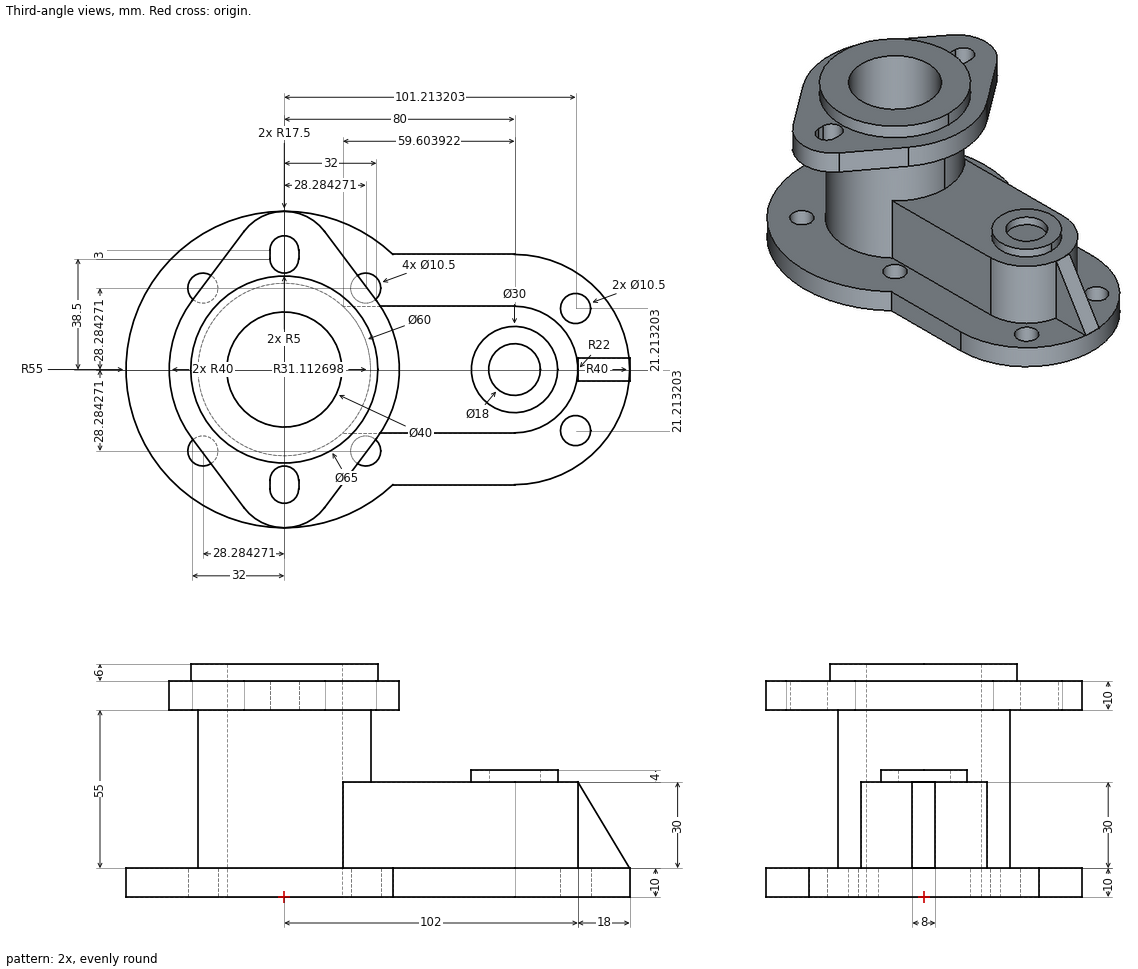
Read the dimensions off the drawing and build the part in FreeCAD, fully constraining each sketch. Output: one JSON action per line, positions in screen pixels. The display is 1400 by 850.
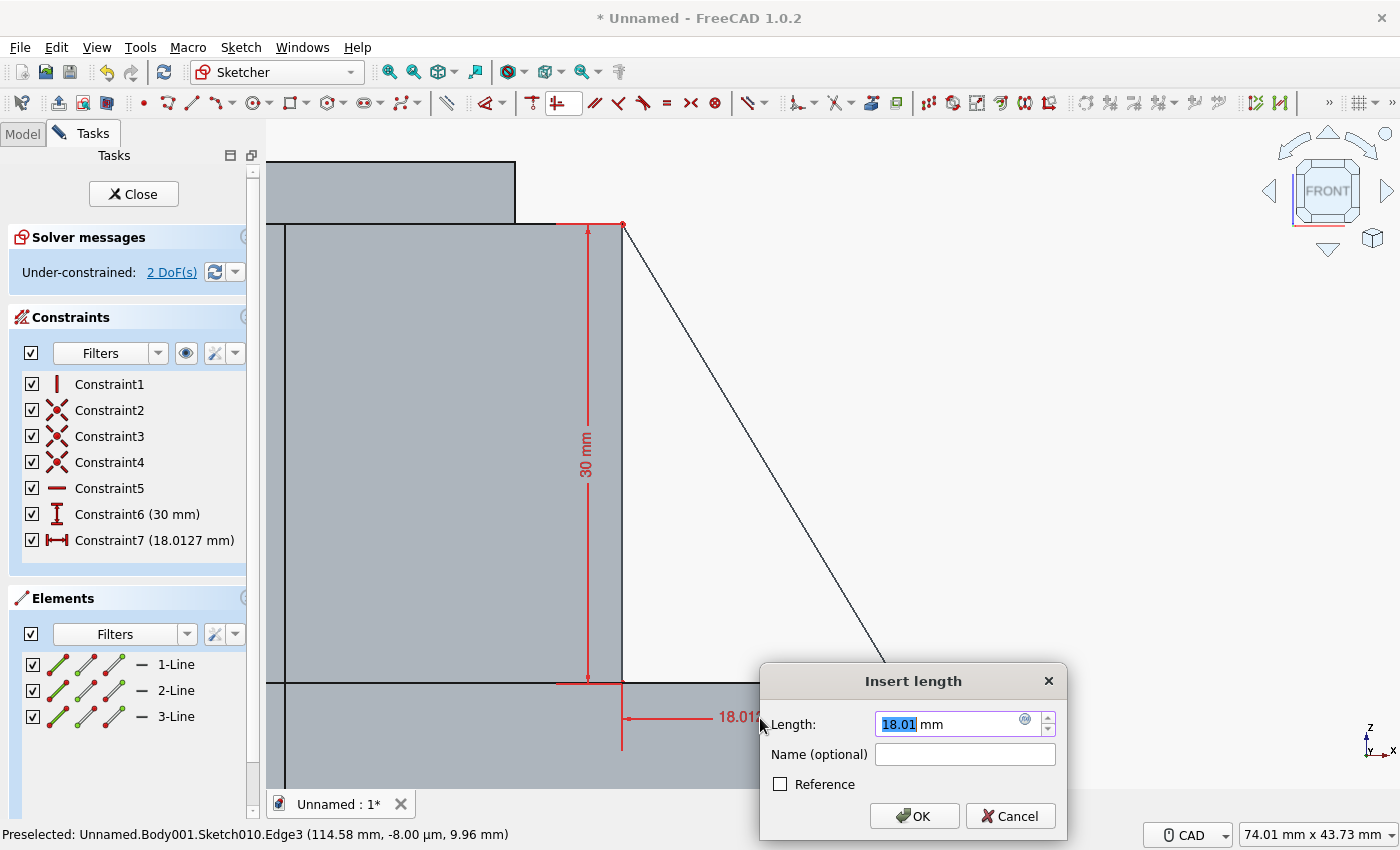
{"action": "type", "text": "18"}
{"action": "key", "text": "Return"}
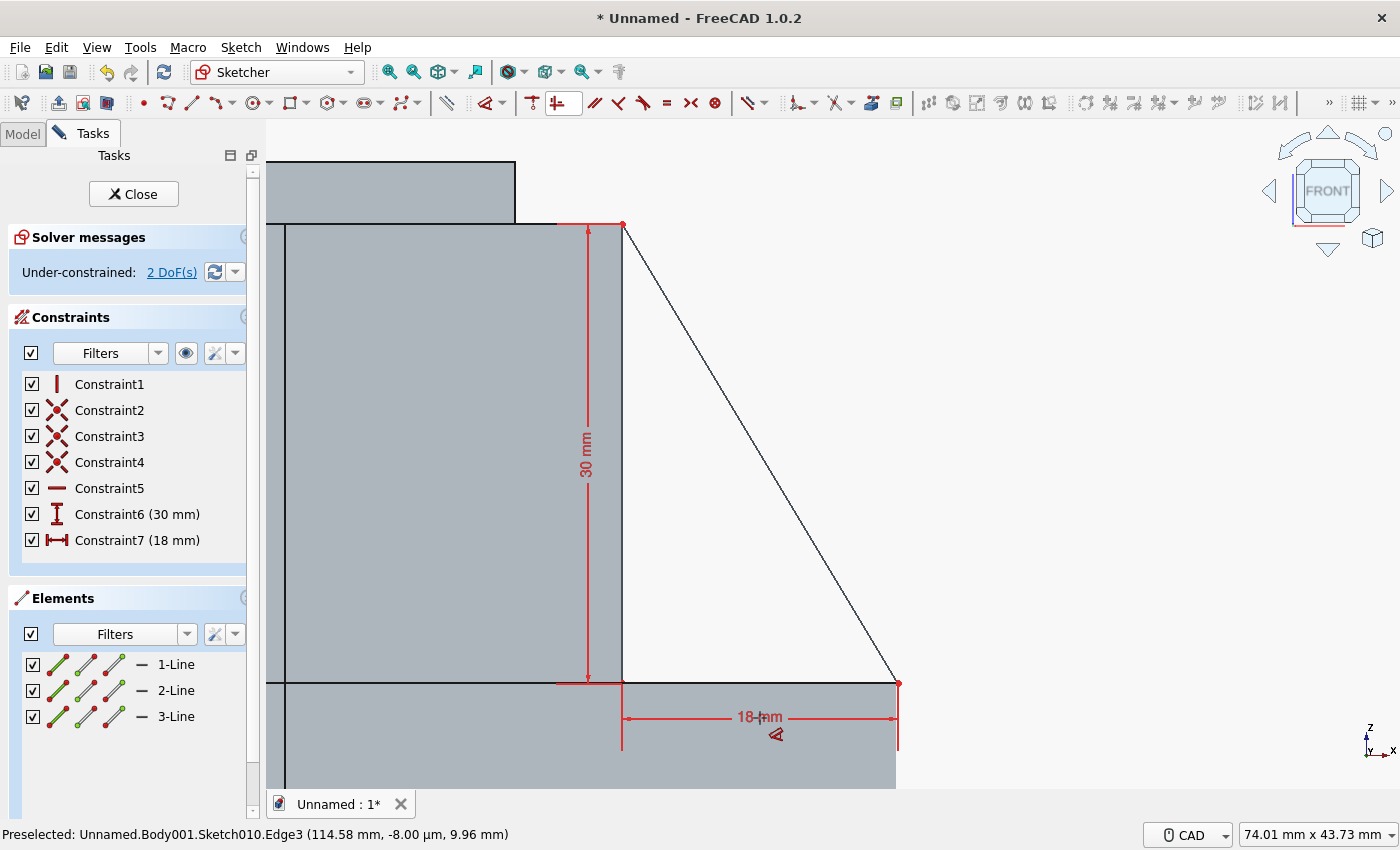
{"action": "left_click", "coordinate": [622, 684]}
{"action": "left_click", "coordinate": [656, 722]}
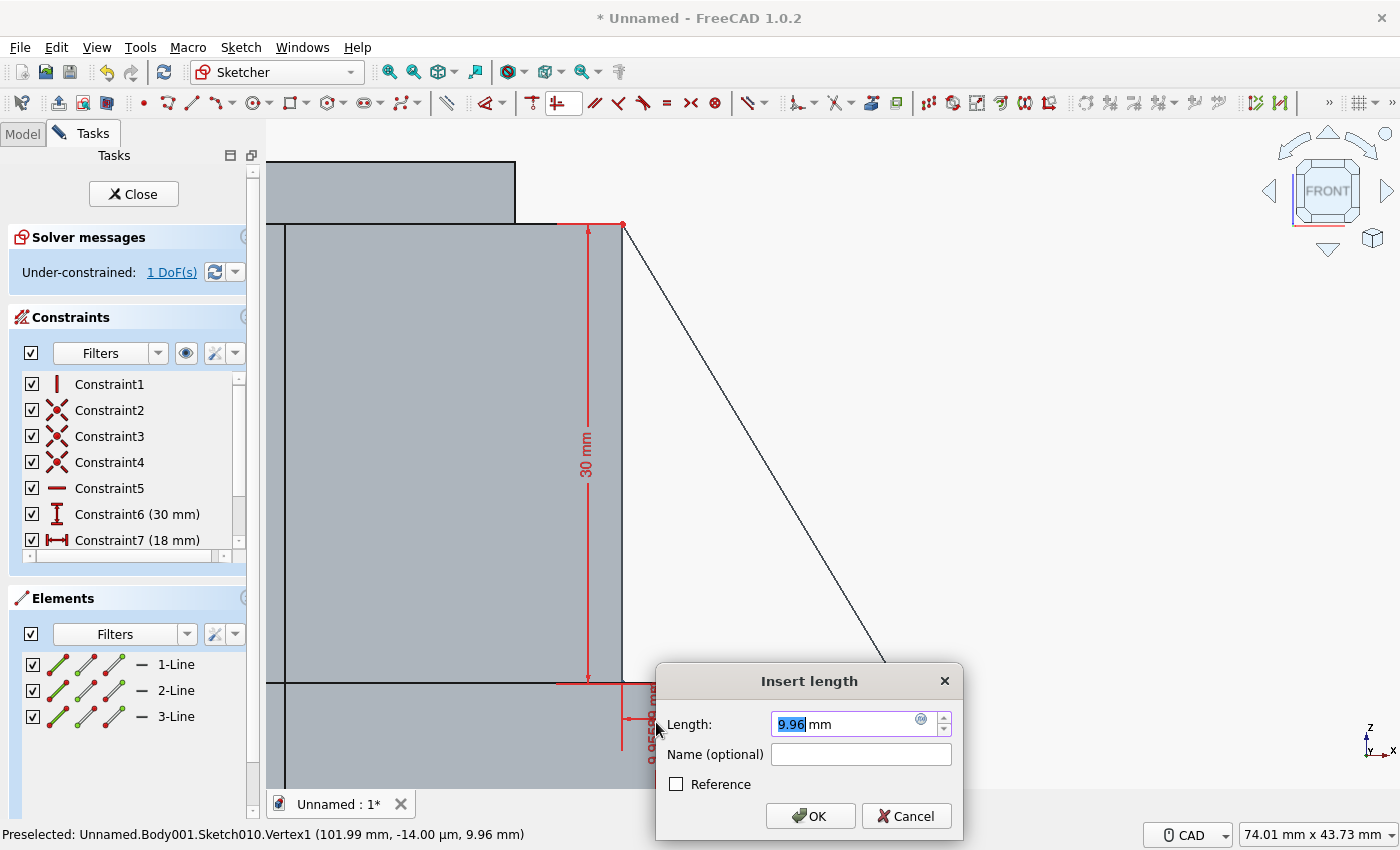
{"action": "type", "text": "10"}
{"action": "key", "text": "Return"}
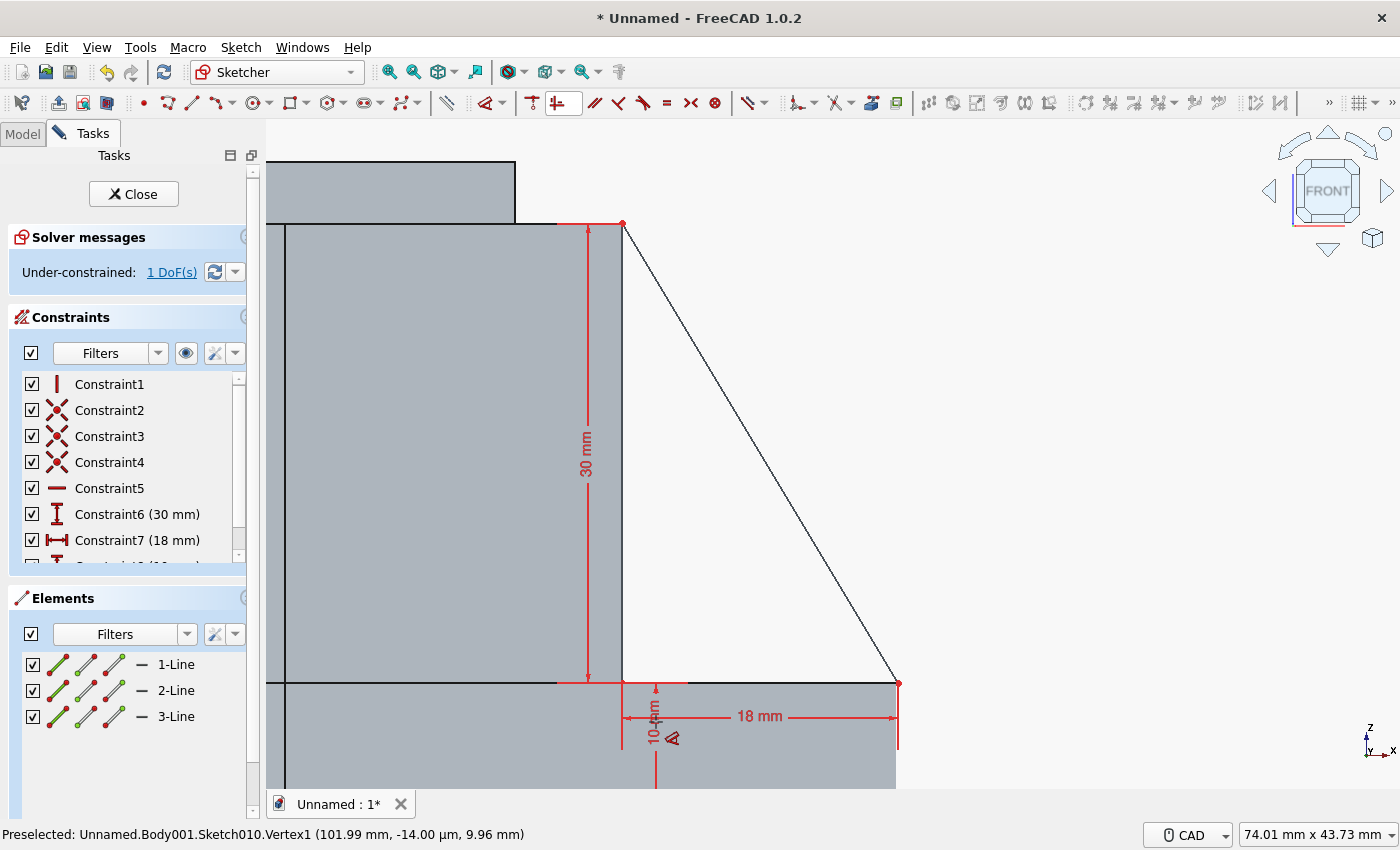
{"action": "left_click", "coordinate": [622, 683]}
{"action": "left_click", "coordinate": [458, 649]}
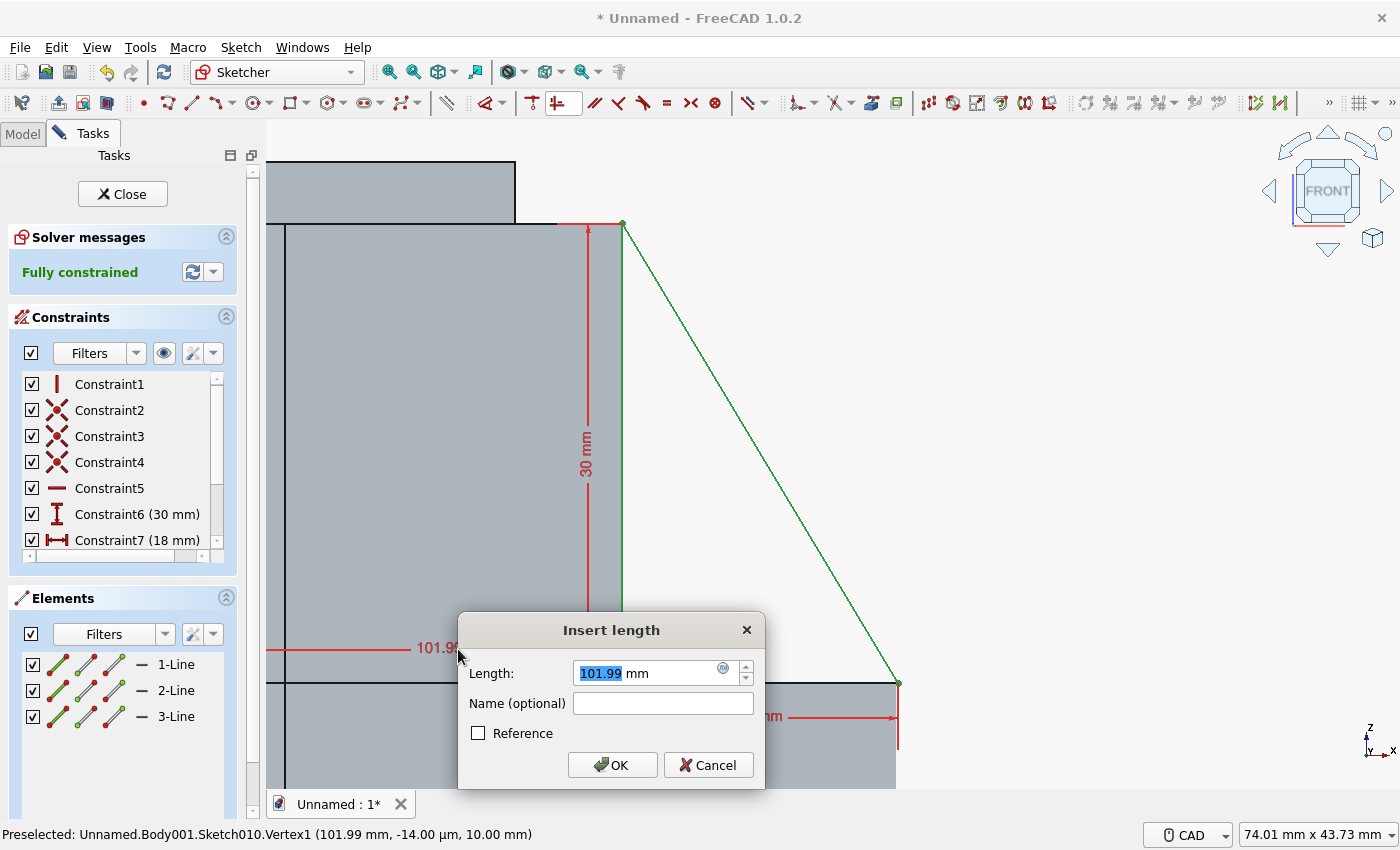
{"action": "type", "text": "102"}
{"action": "key", "text": "Return"}
{"action": "key", "text": "Escape"}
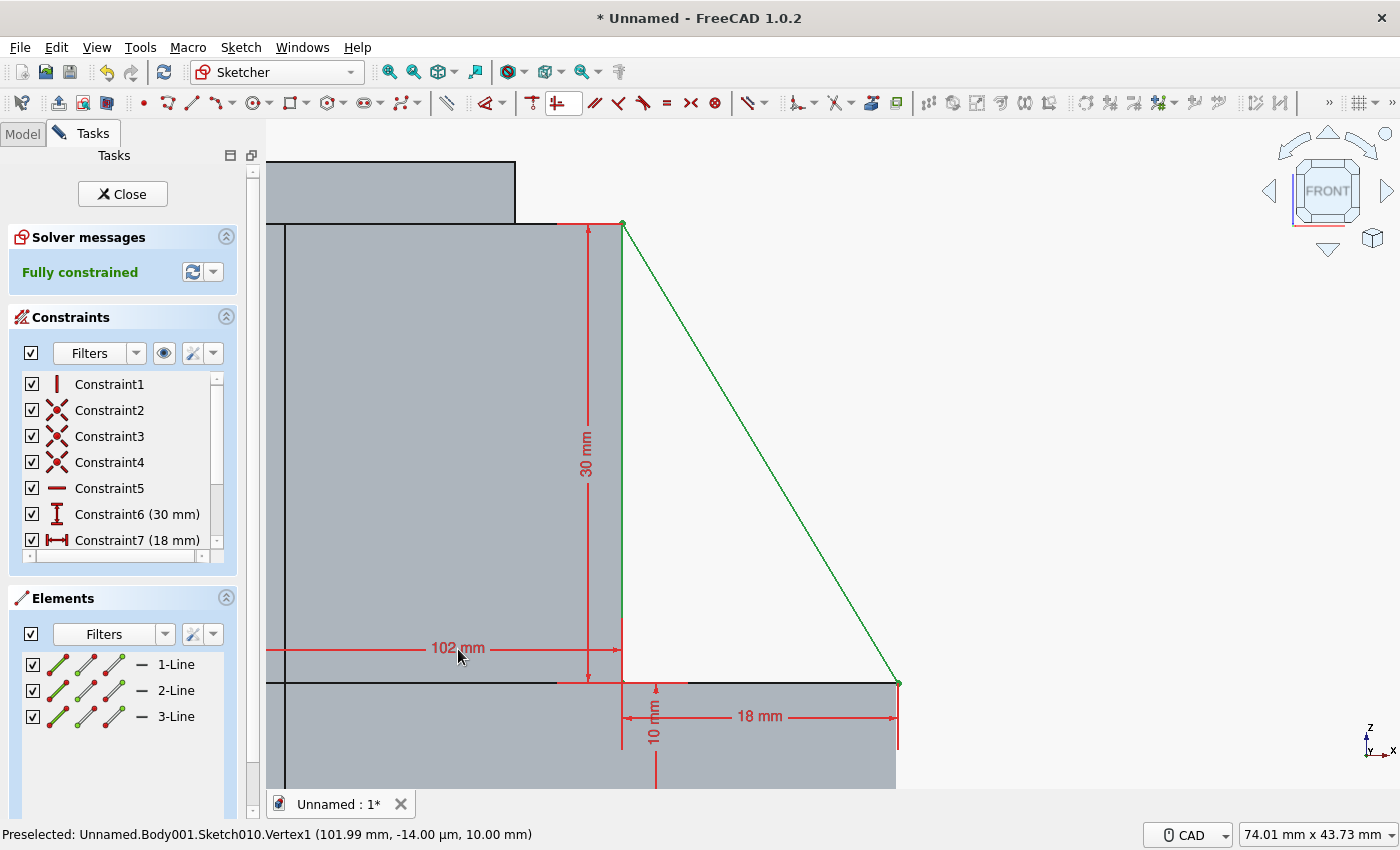
{"action": "left_click", "coordinate": [123, 194]}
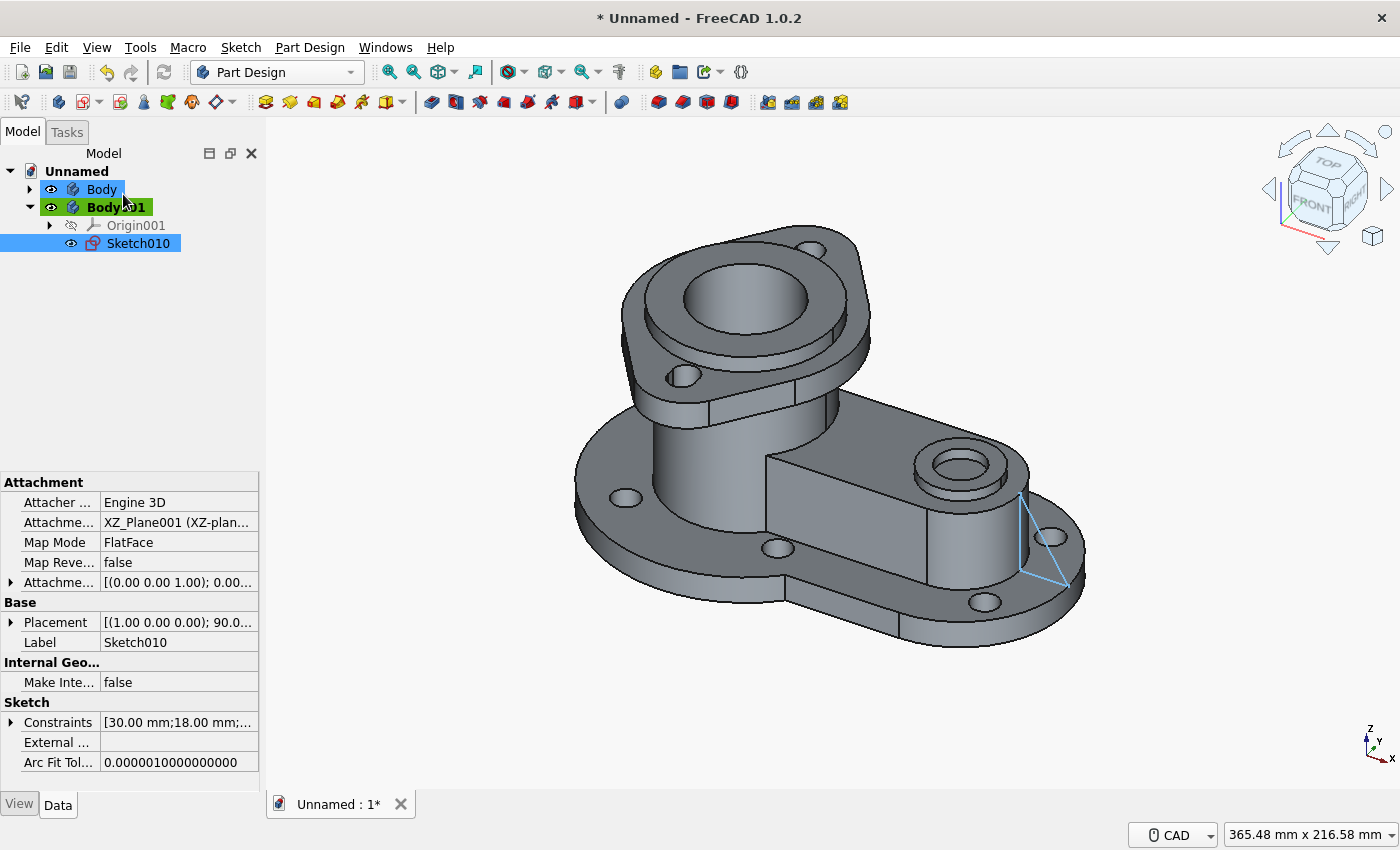
{"action": "left_click", "coordinate": [266, 102]}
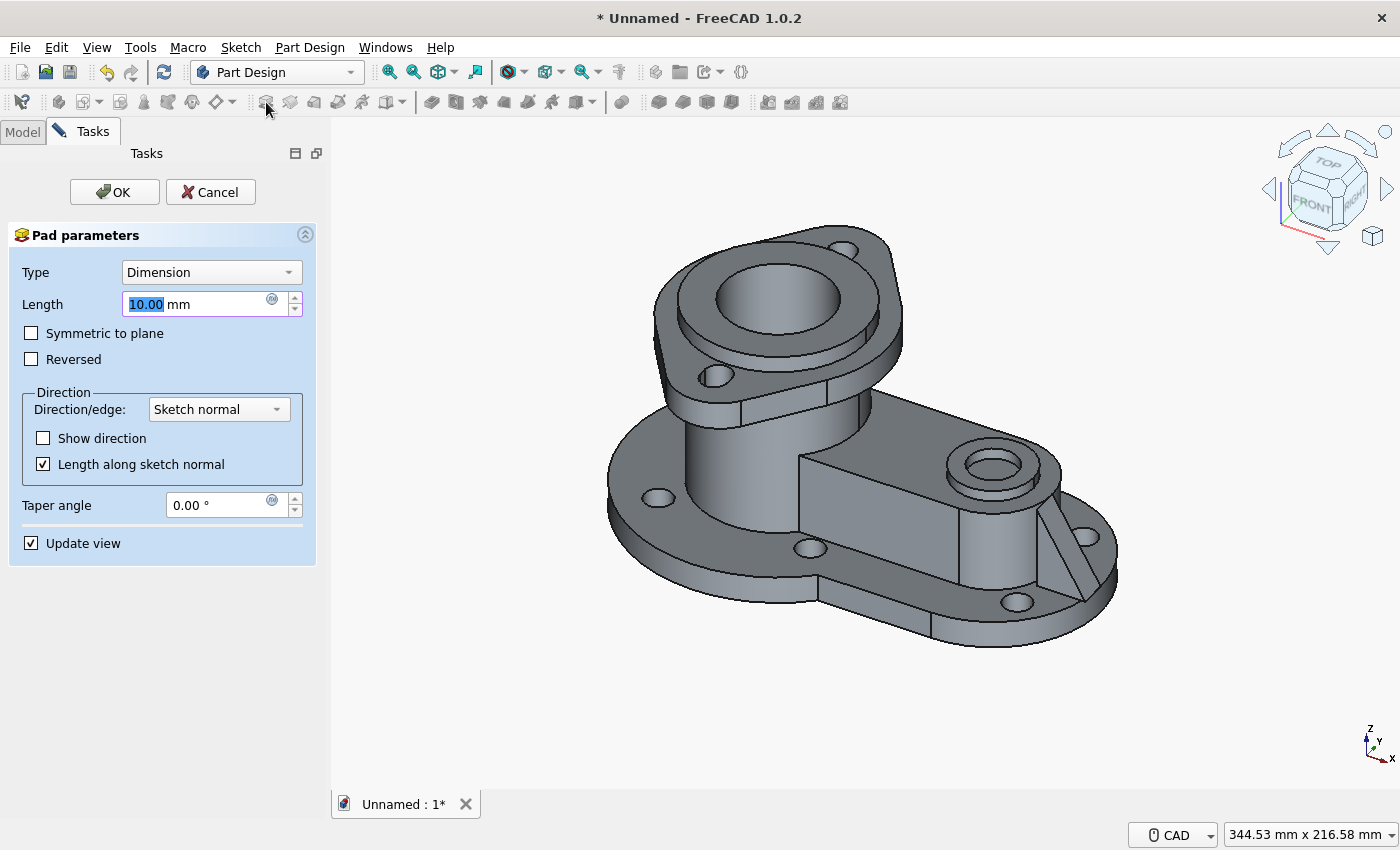
{"action": "type", "text": "8"}
{"action": "key", "text": "Tab"}